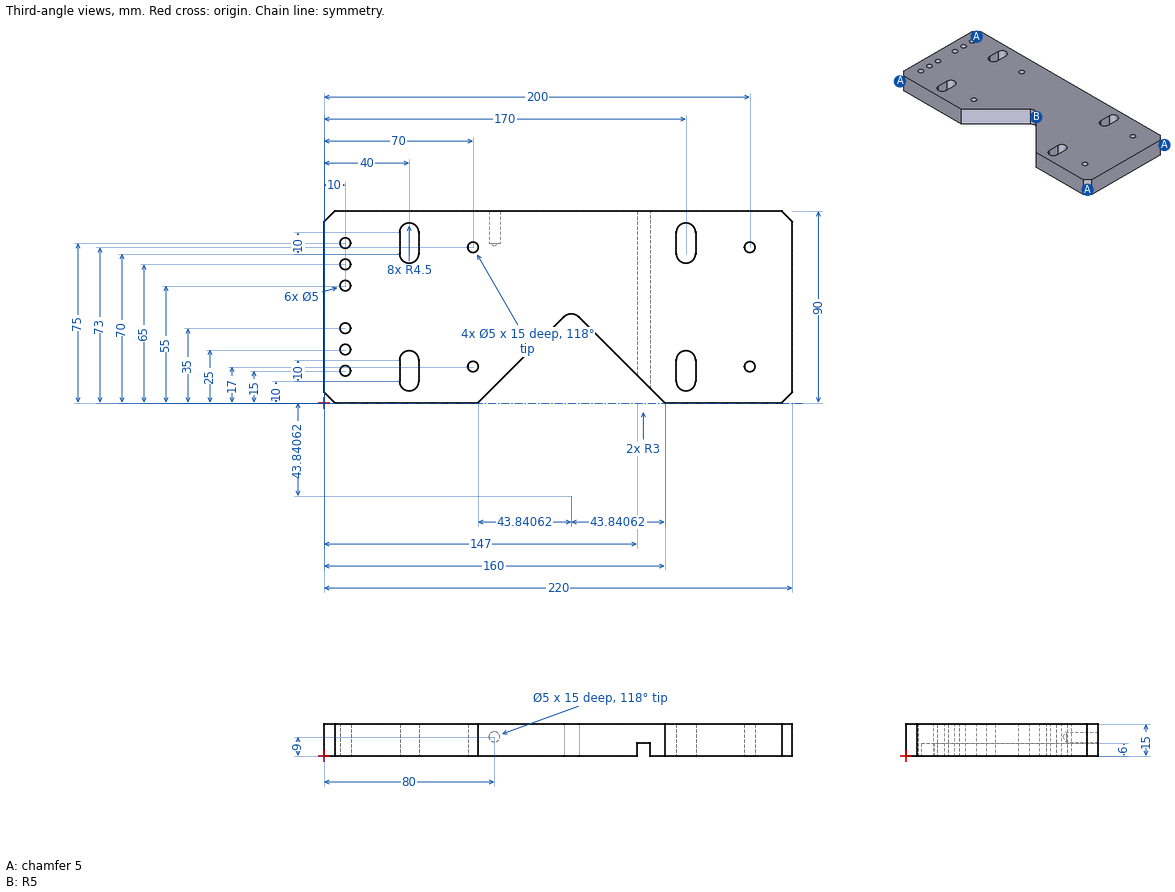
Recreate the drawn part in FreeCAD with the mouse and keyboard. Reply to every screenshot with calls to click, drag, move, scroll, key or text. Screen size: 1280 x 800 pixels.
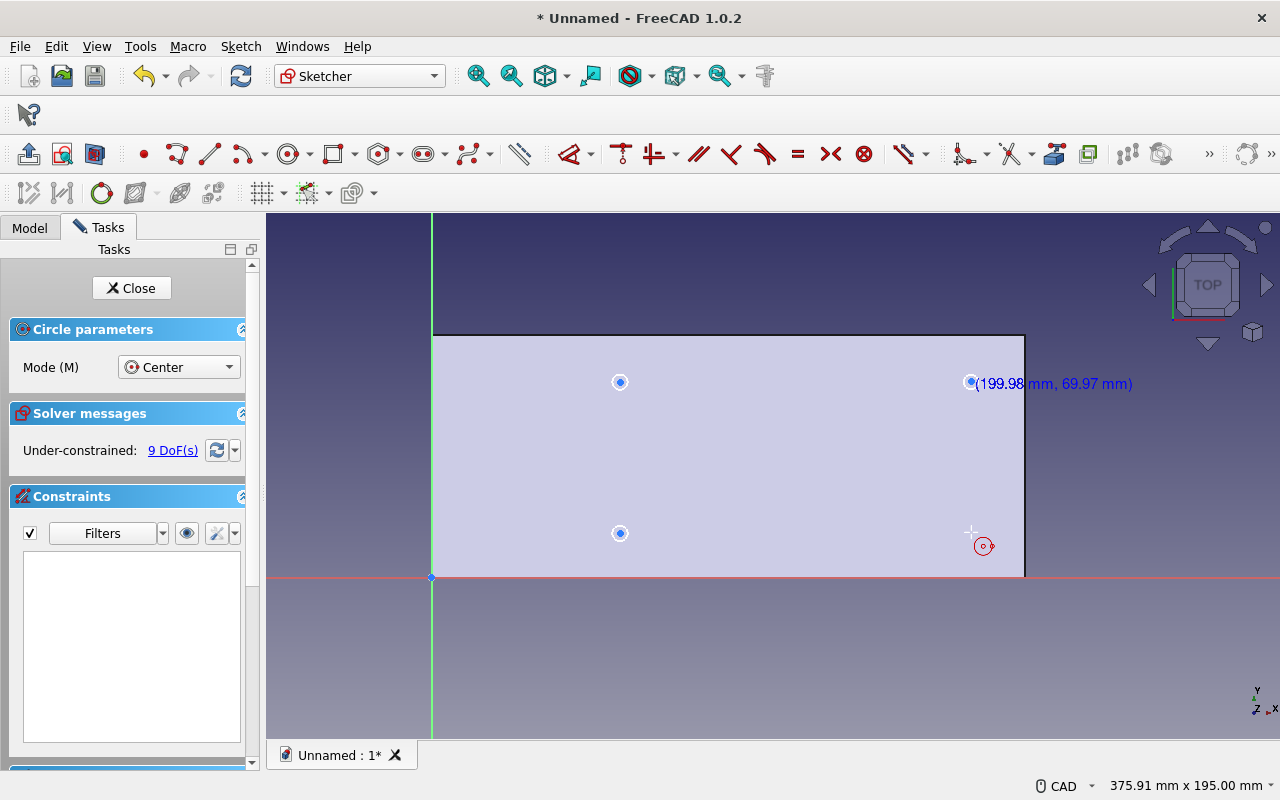
click(971, 532)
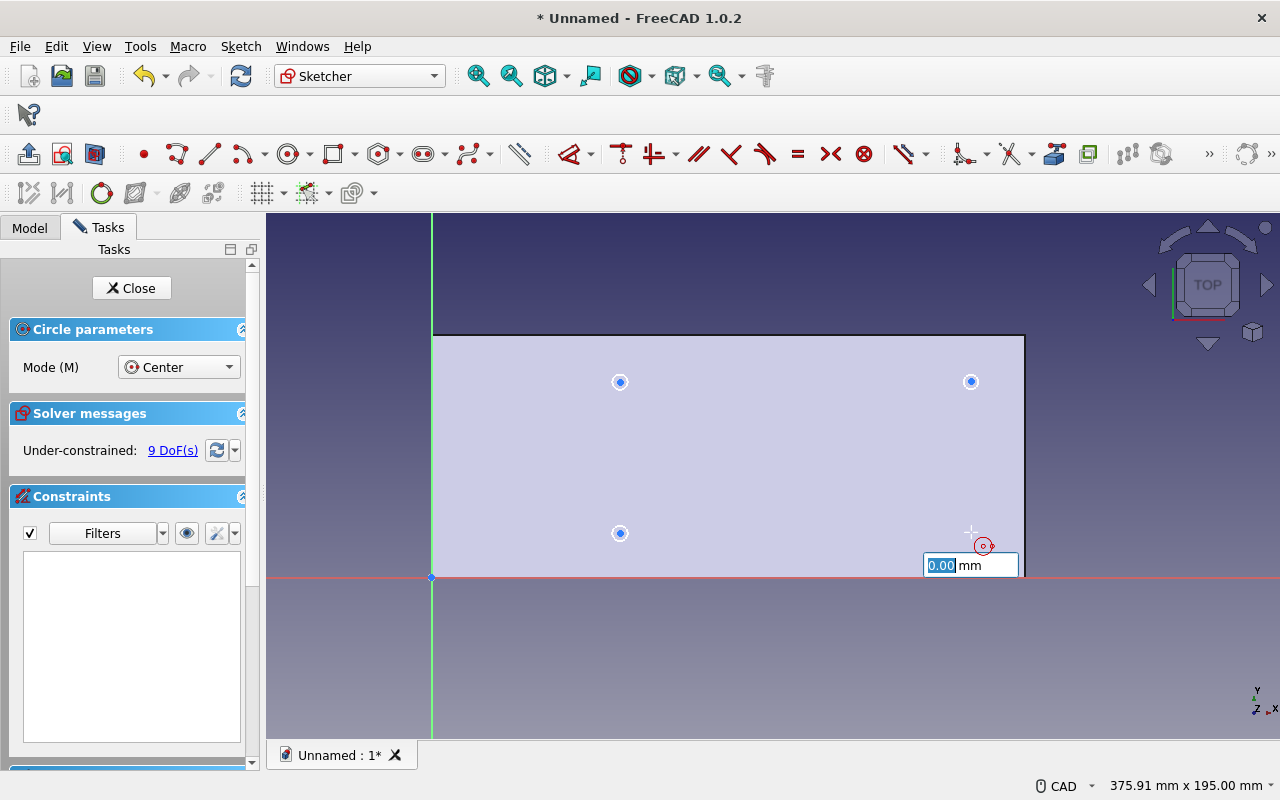
scroll(976, 527, up, 5)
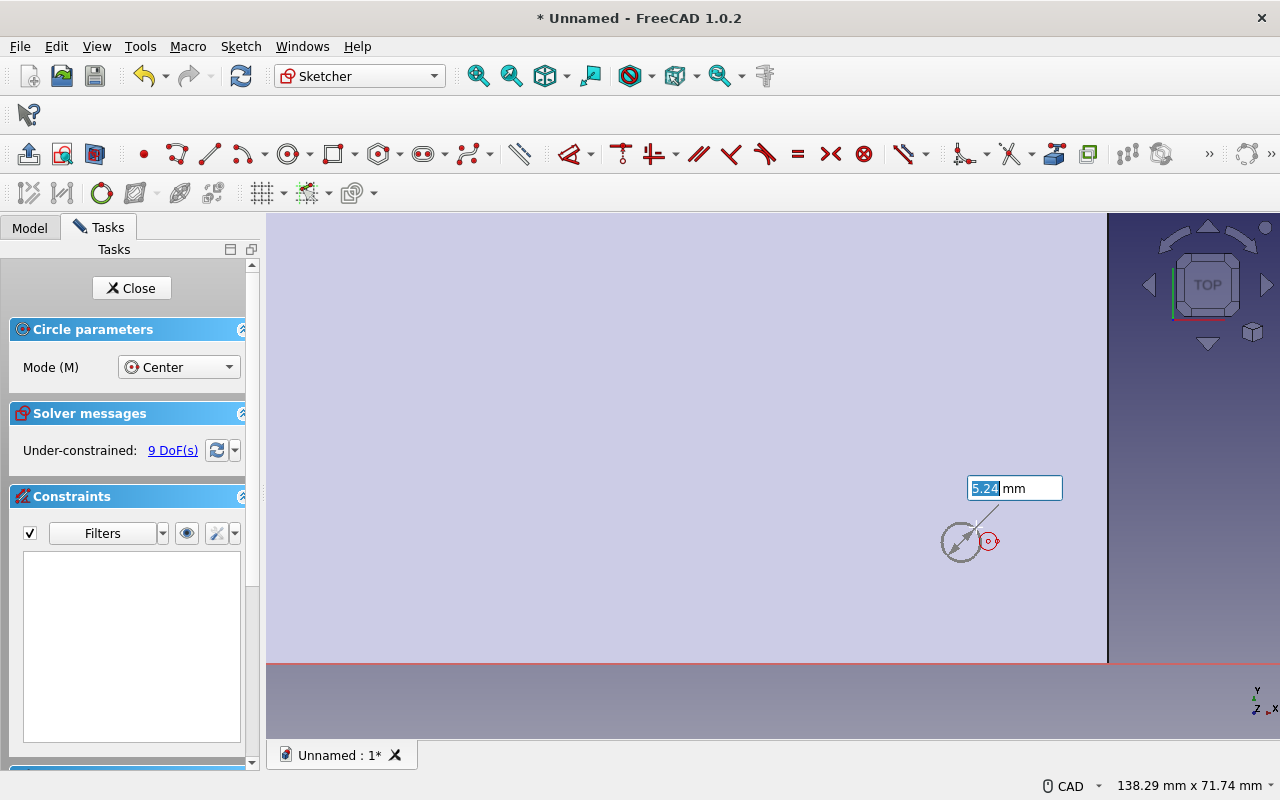
click(974, 527)
key(Escape)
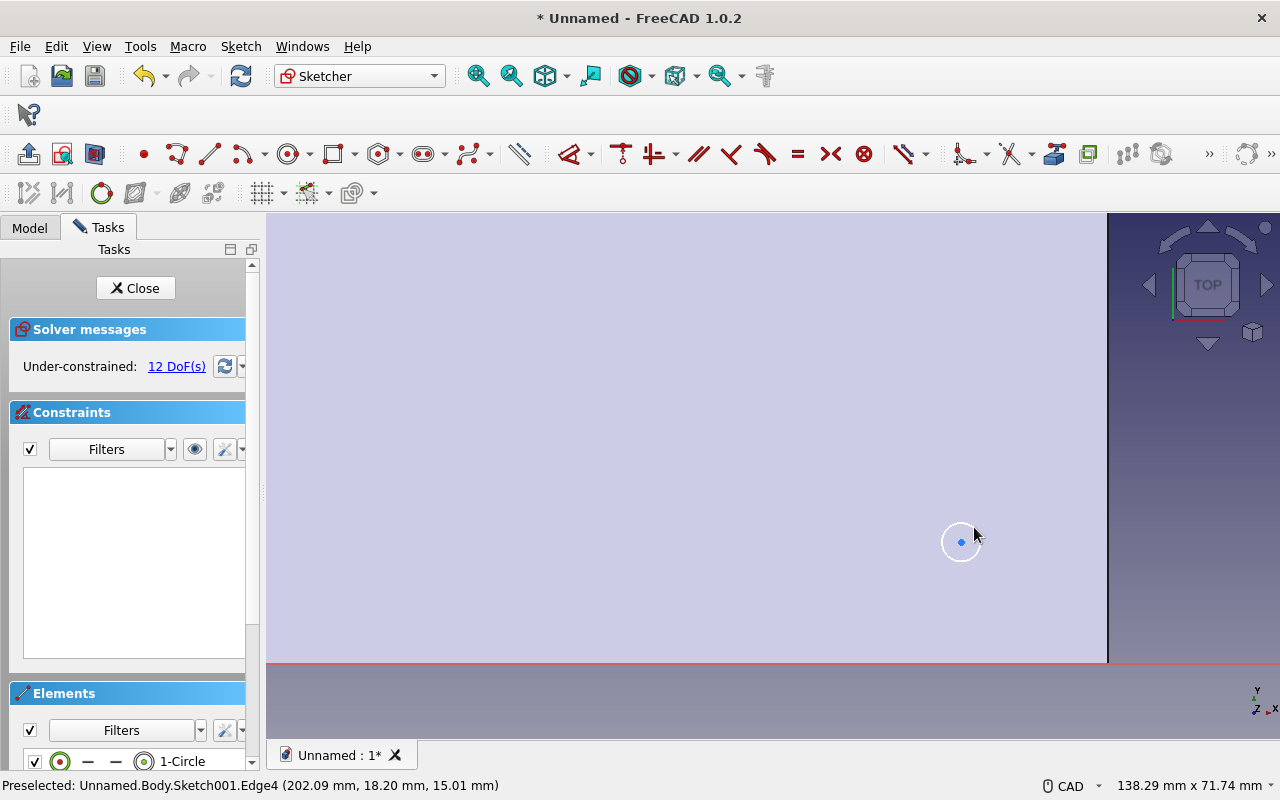
scroll(976, 527, down, 5)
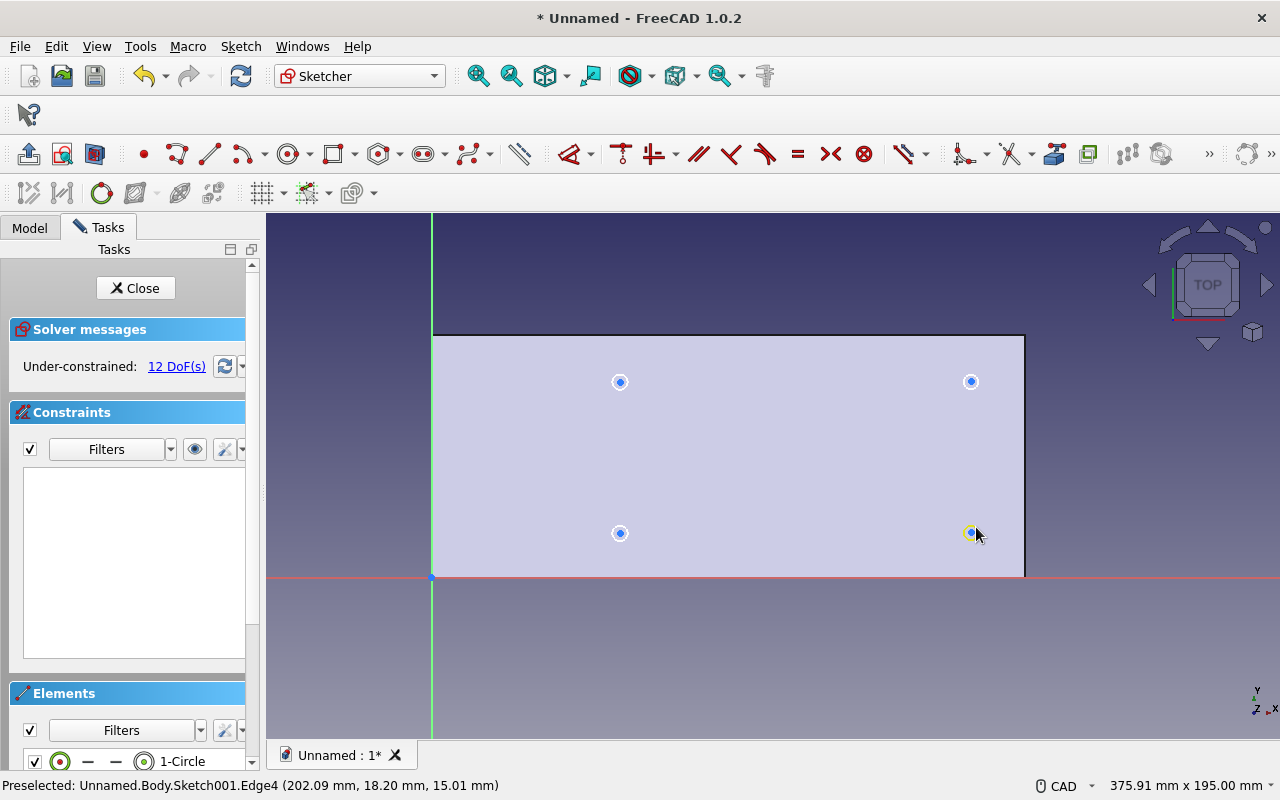
scroll(625, 377, up, 4)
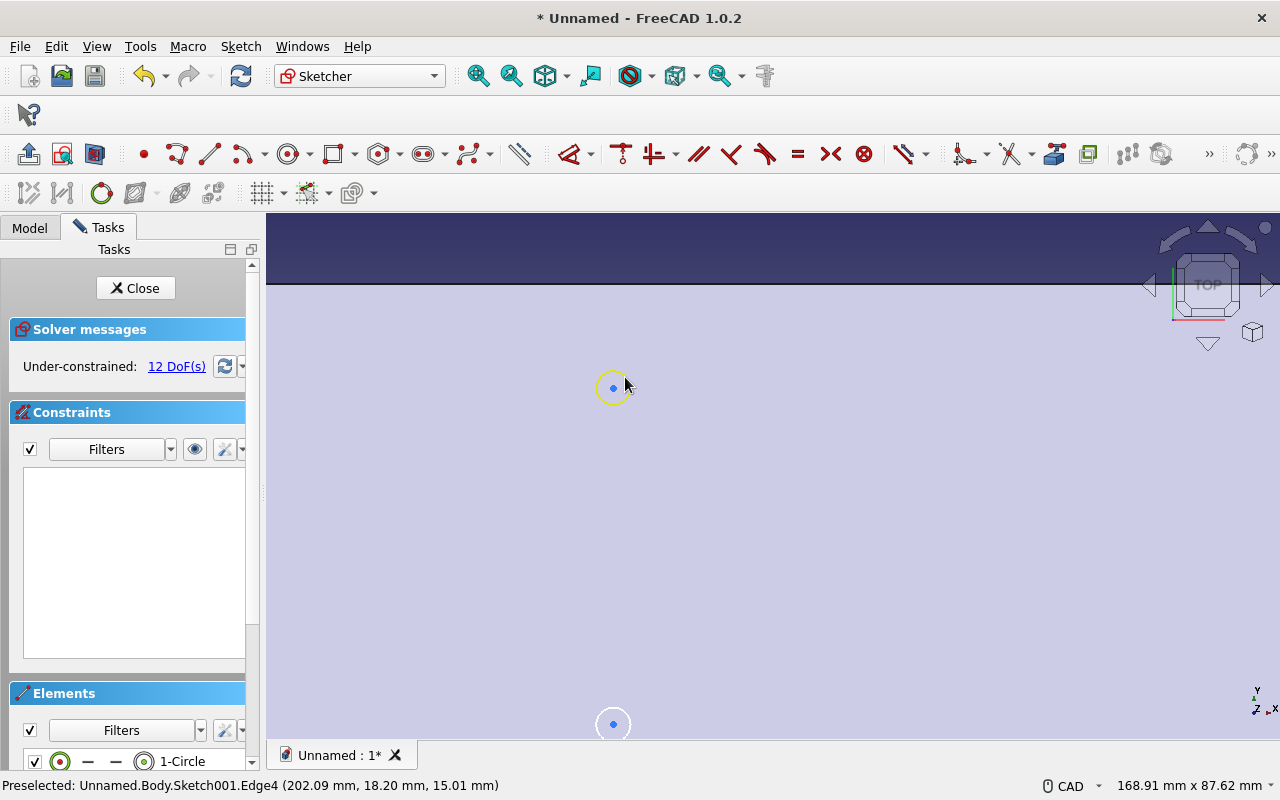
click(625, 376)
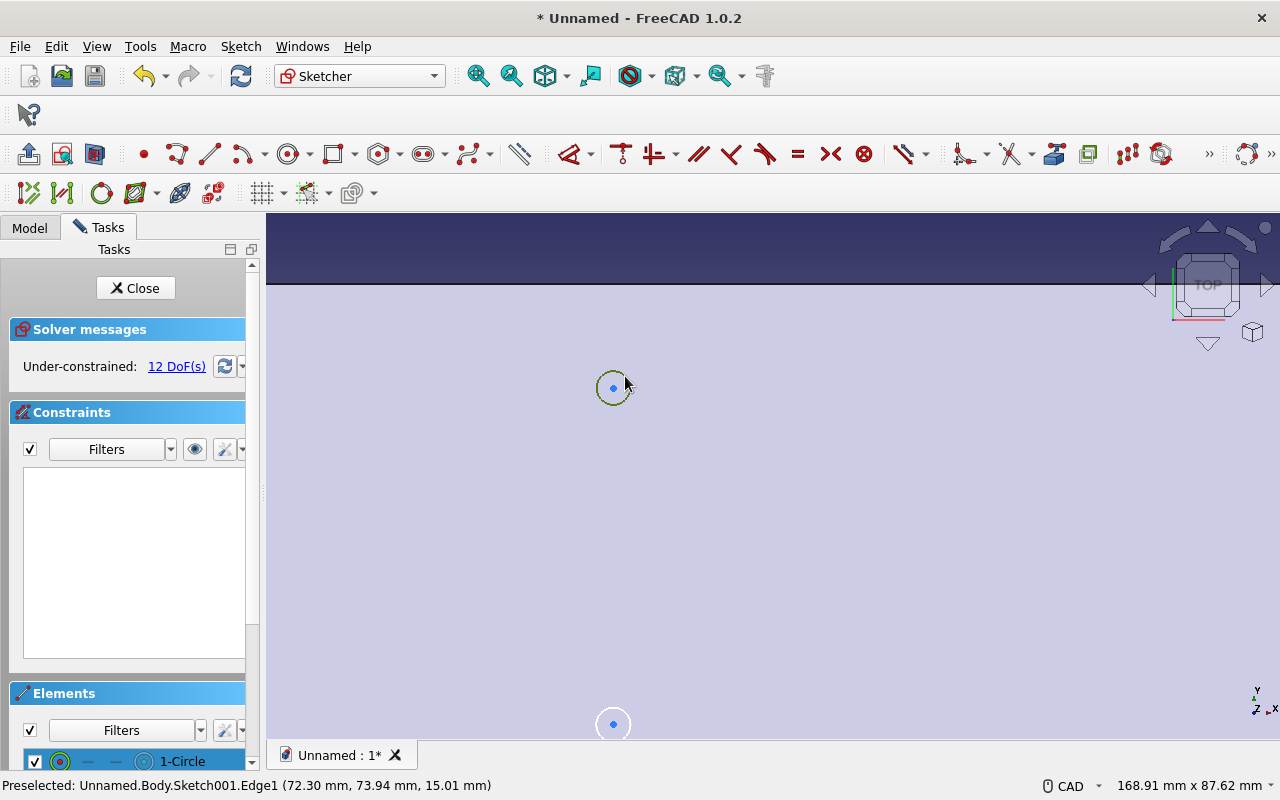
click(614, 708)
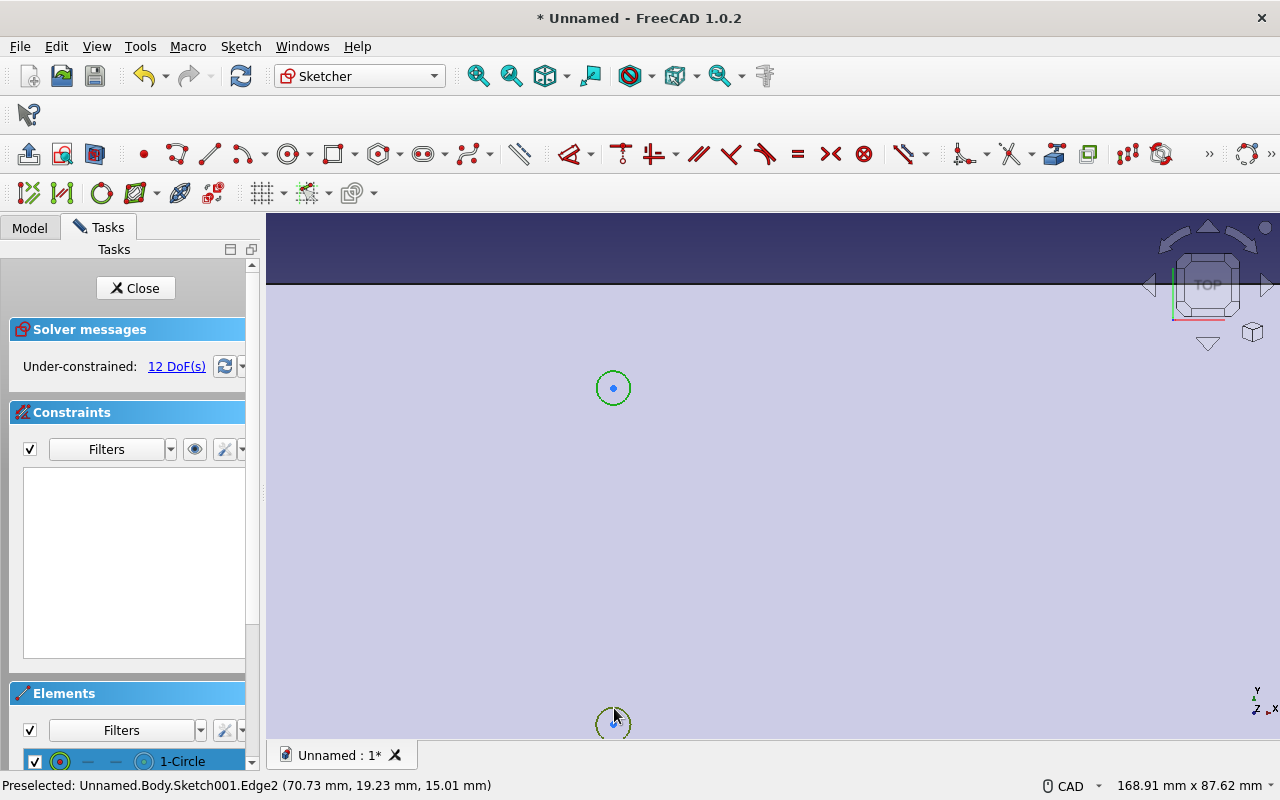
scroll(625, 377, down, 4)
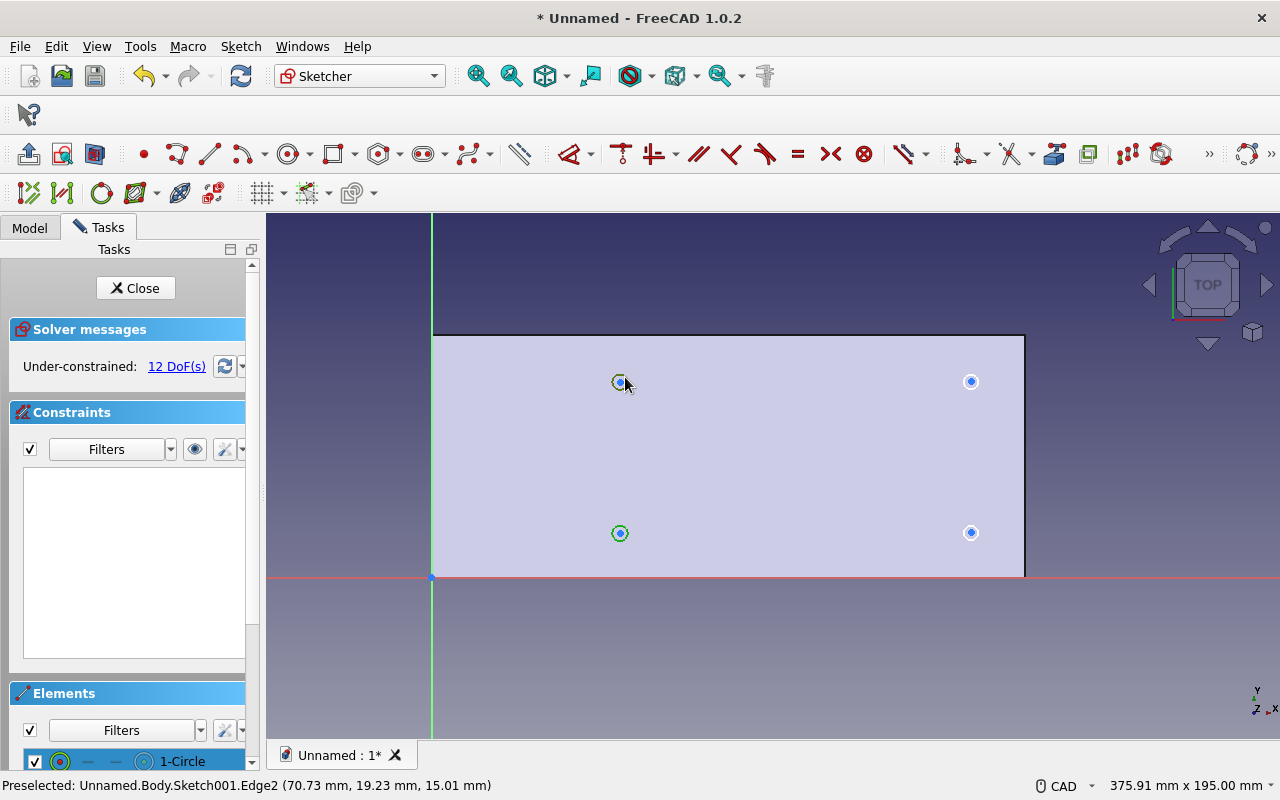
scroll(976, 377, up, 4)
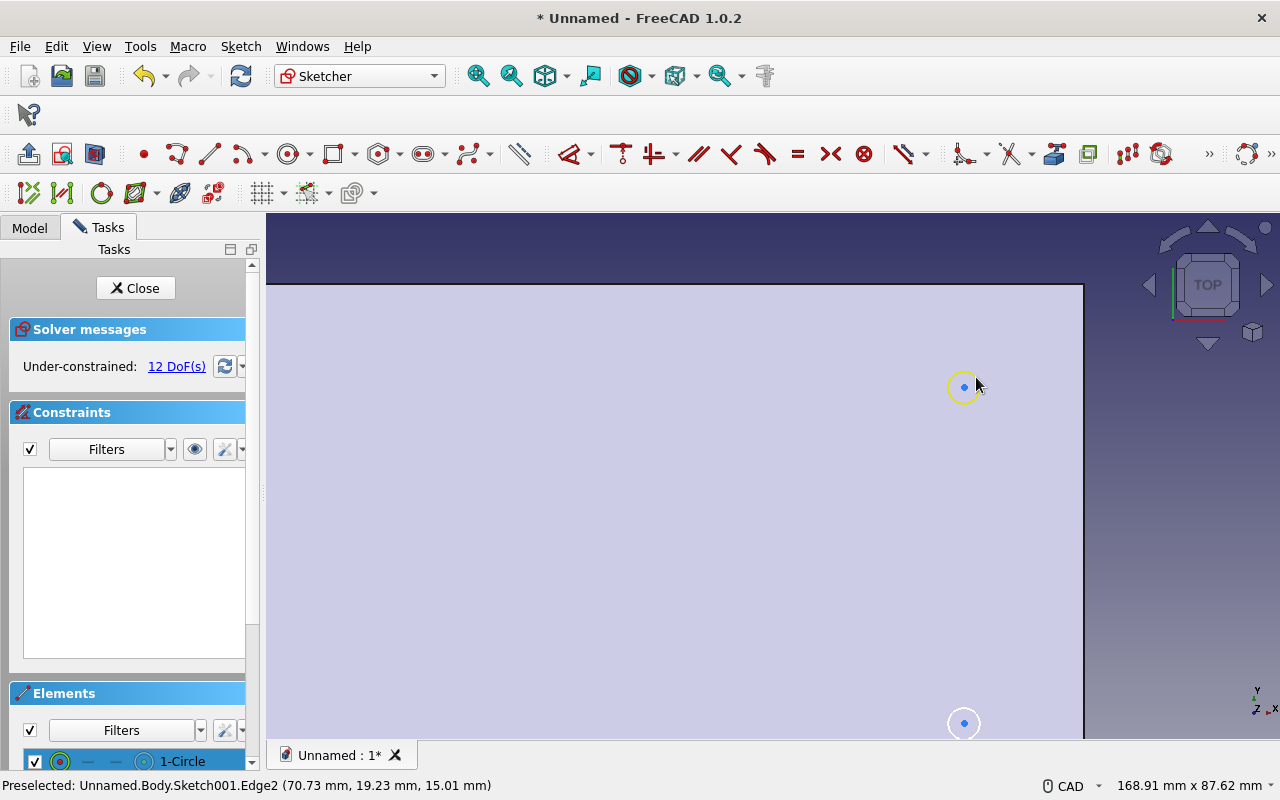
click(975, 376)